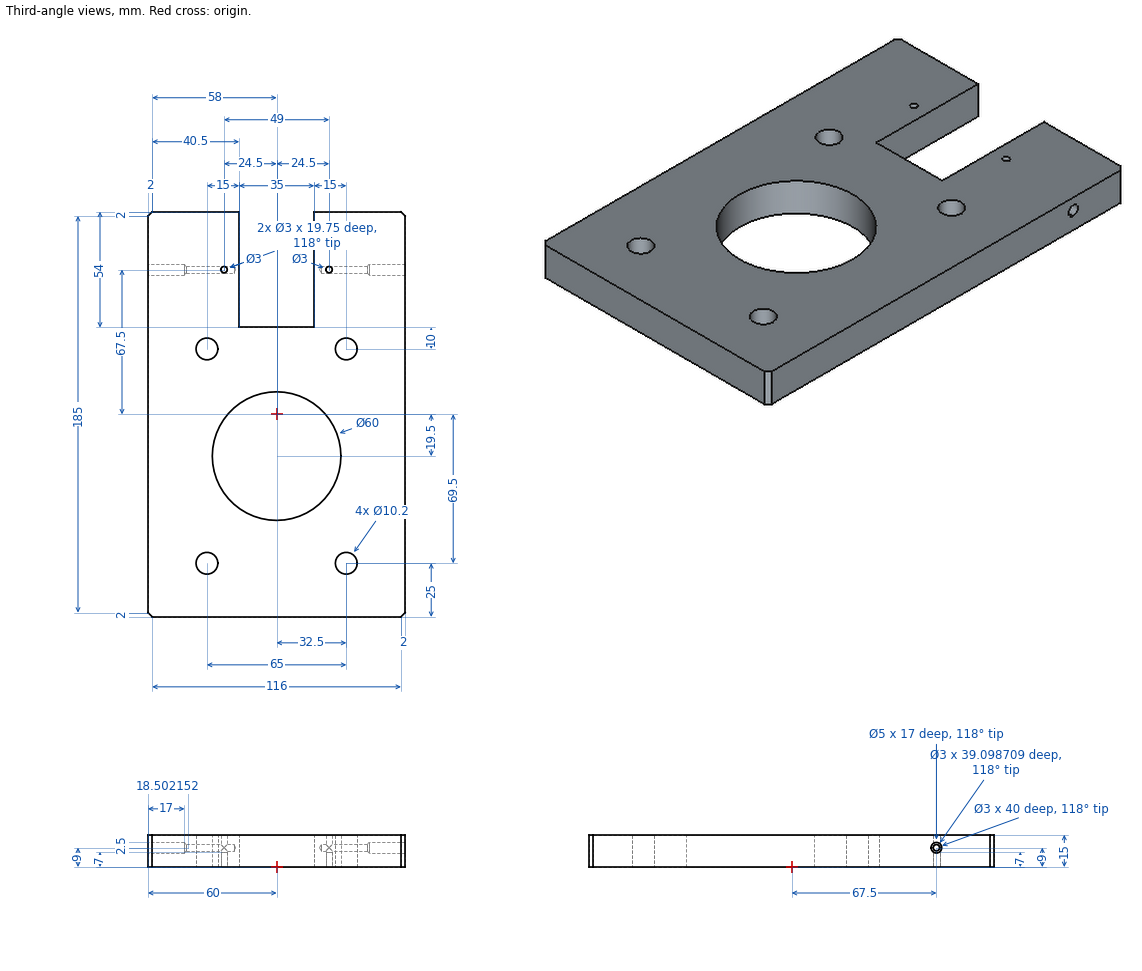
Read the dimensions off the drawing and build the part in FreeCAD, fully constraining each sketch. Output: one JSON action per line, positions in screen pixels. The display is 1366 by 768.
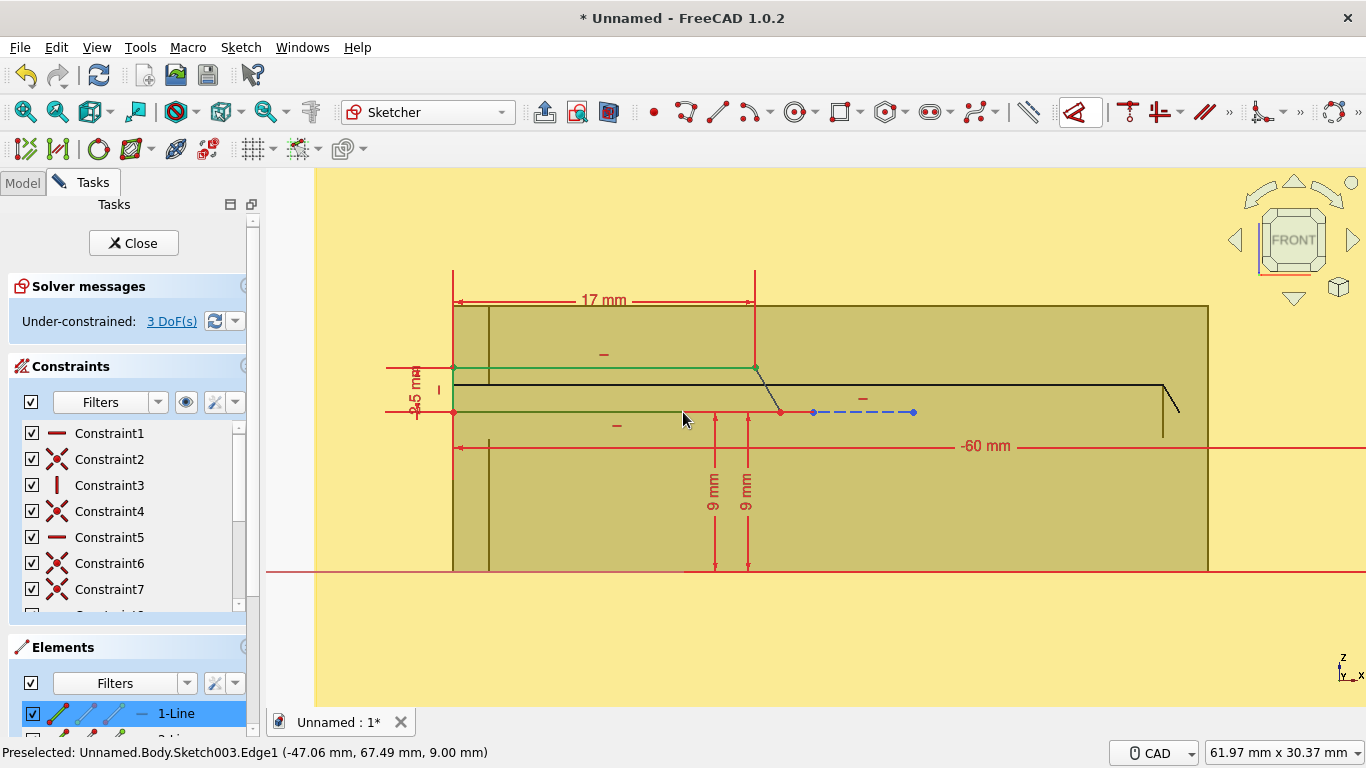
{"action": "key", "text": "l"}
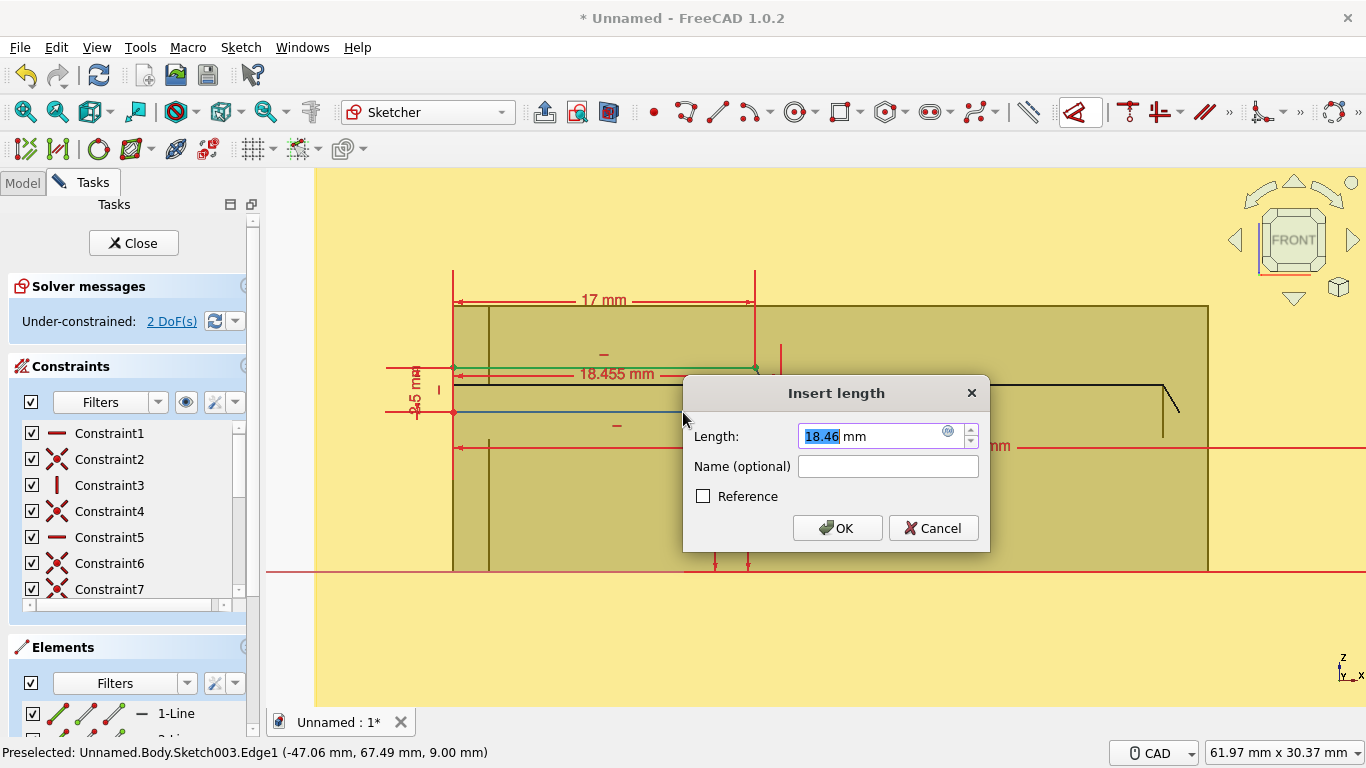
{"action": "type", "text": "18.502152"}
{"action": "key", "text": "Return"}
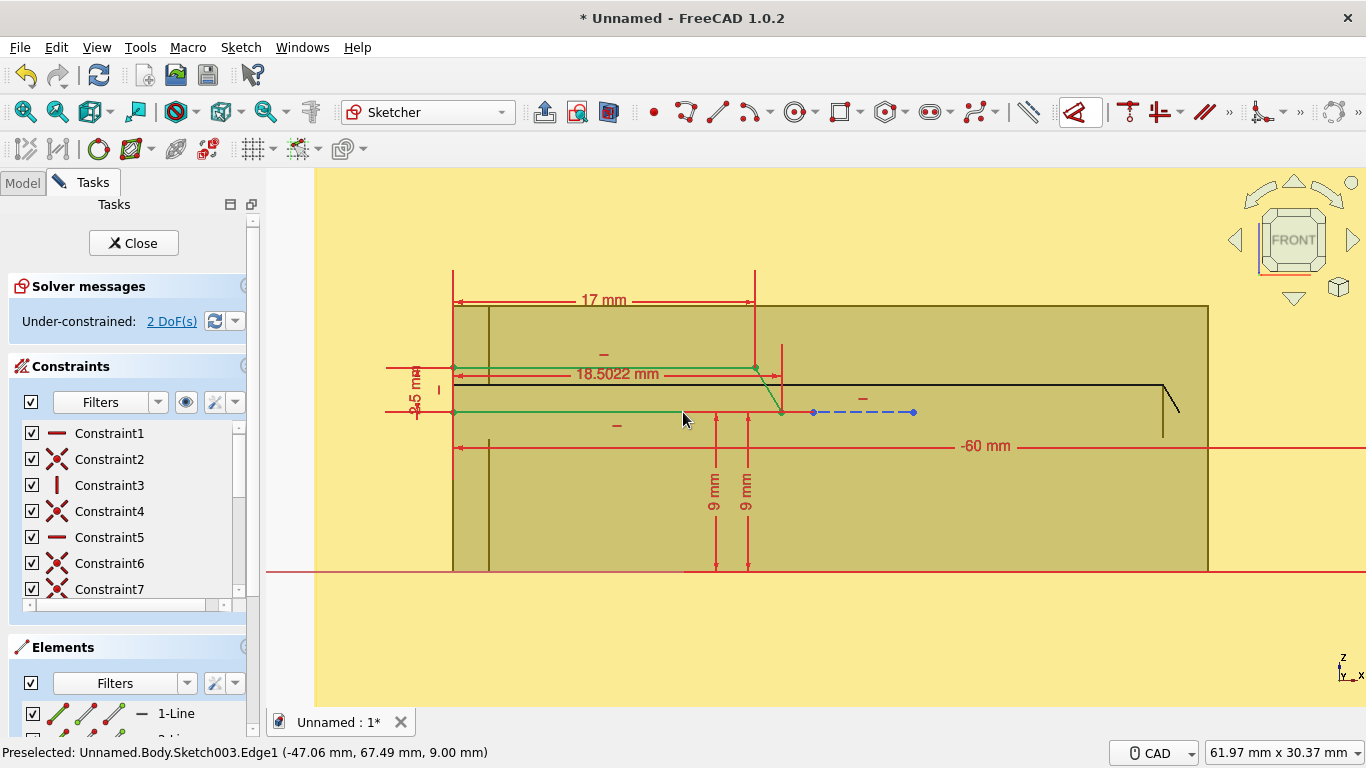
{"action": "left_click", "coordinate": [134, 243]}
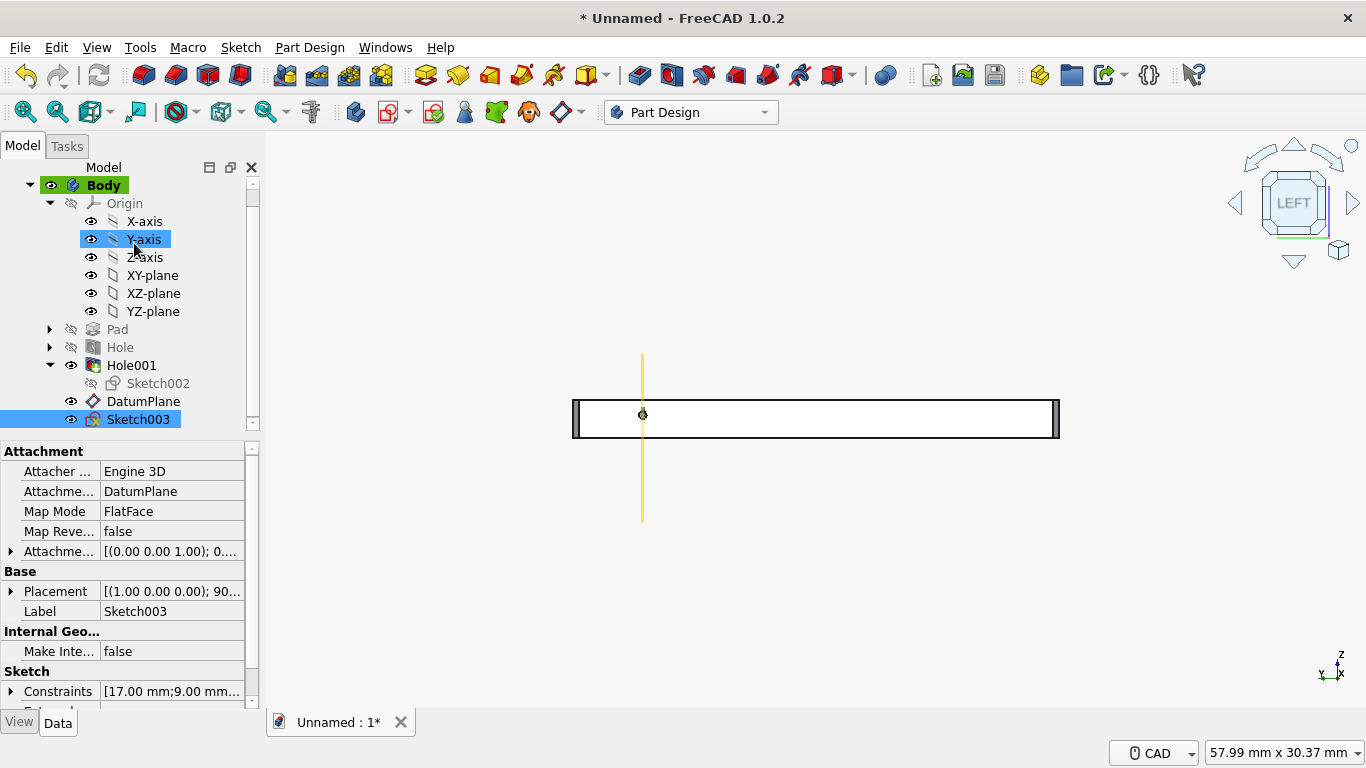
{"action": "left_click", "coordinate": [704, 76]}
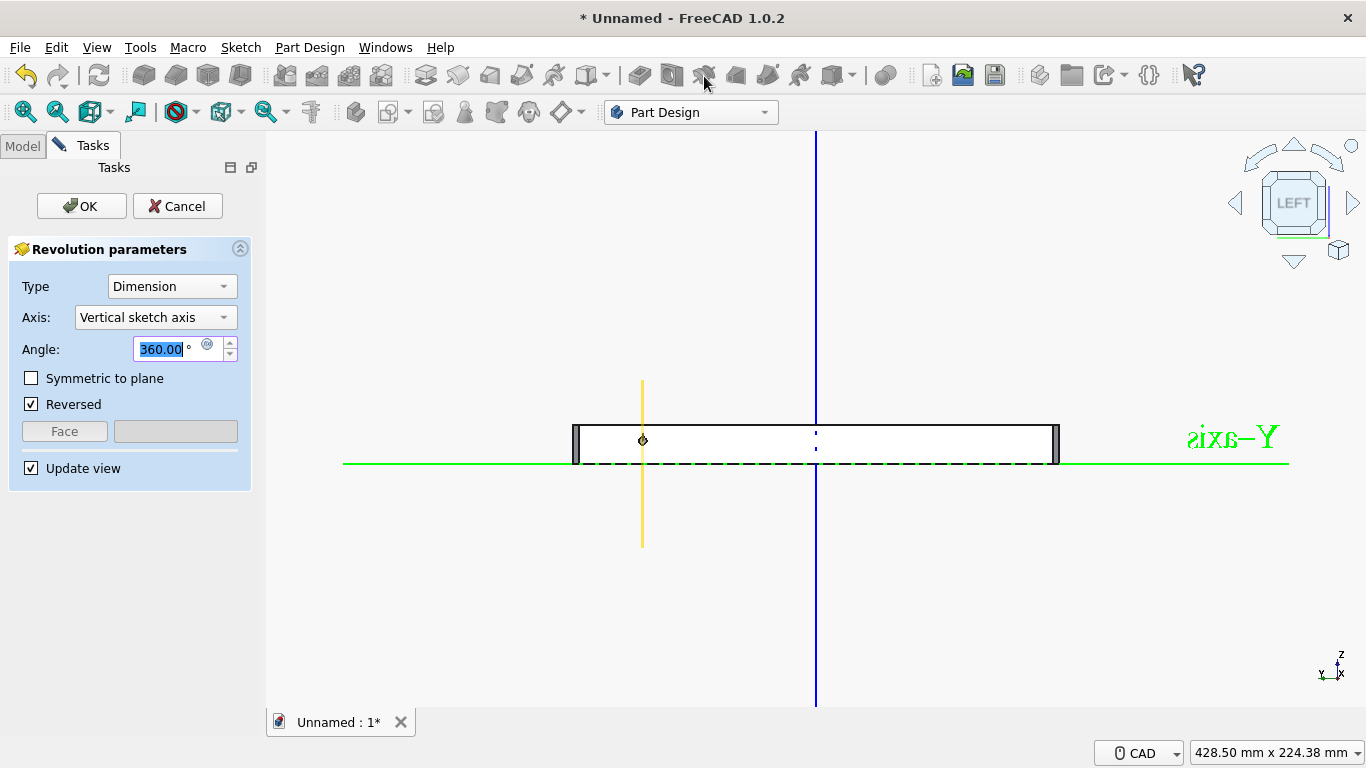
{"action": "left_click", "coordinate": [156, 318]}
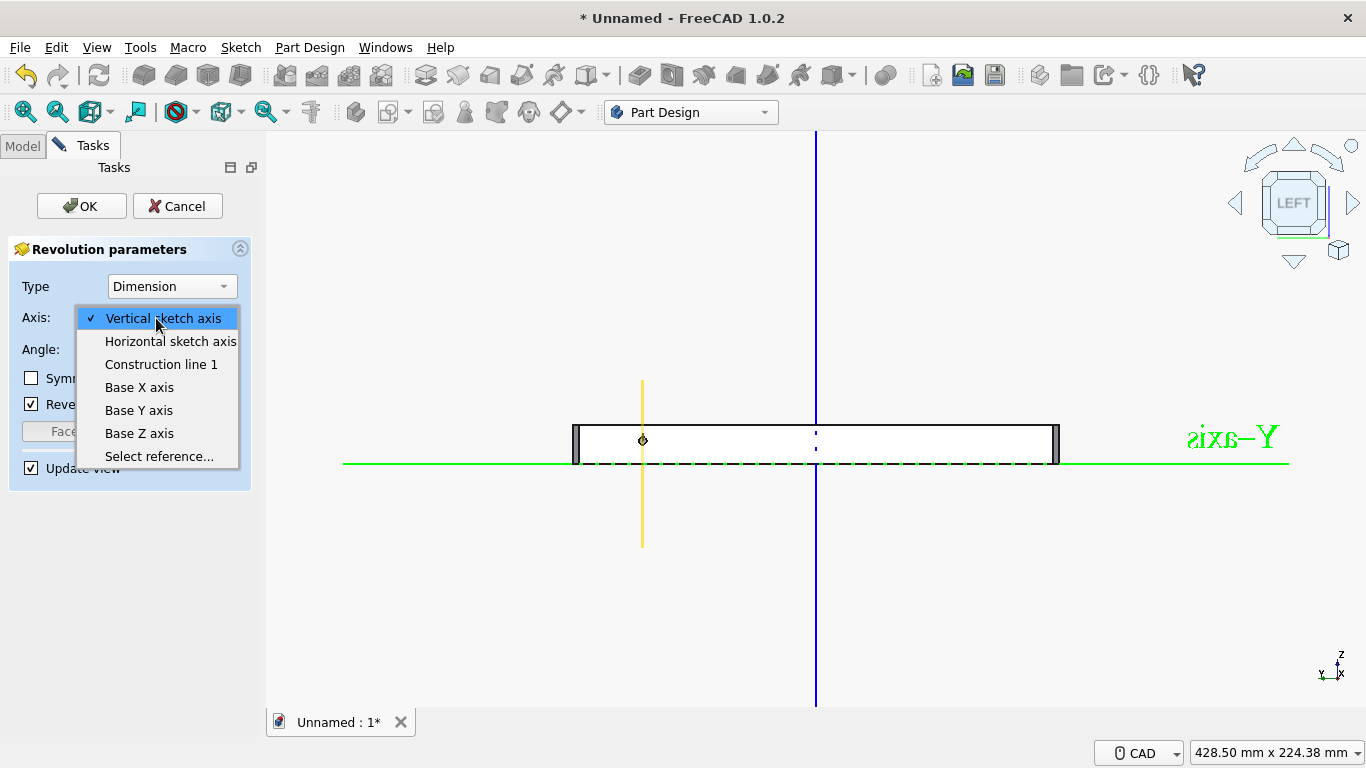
{"action": "left_click", "coordinate": [156, 364]}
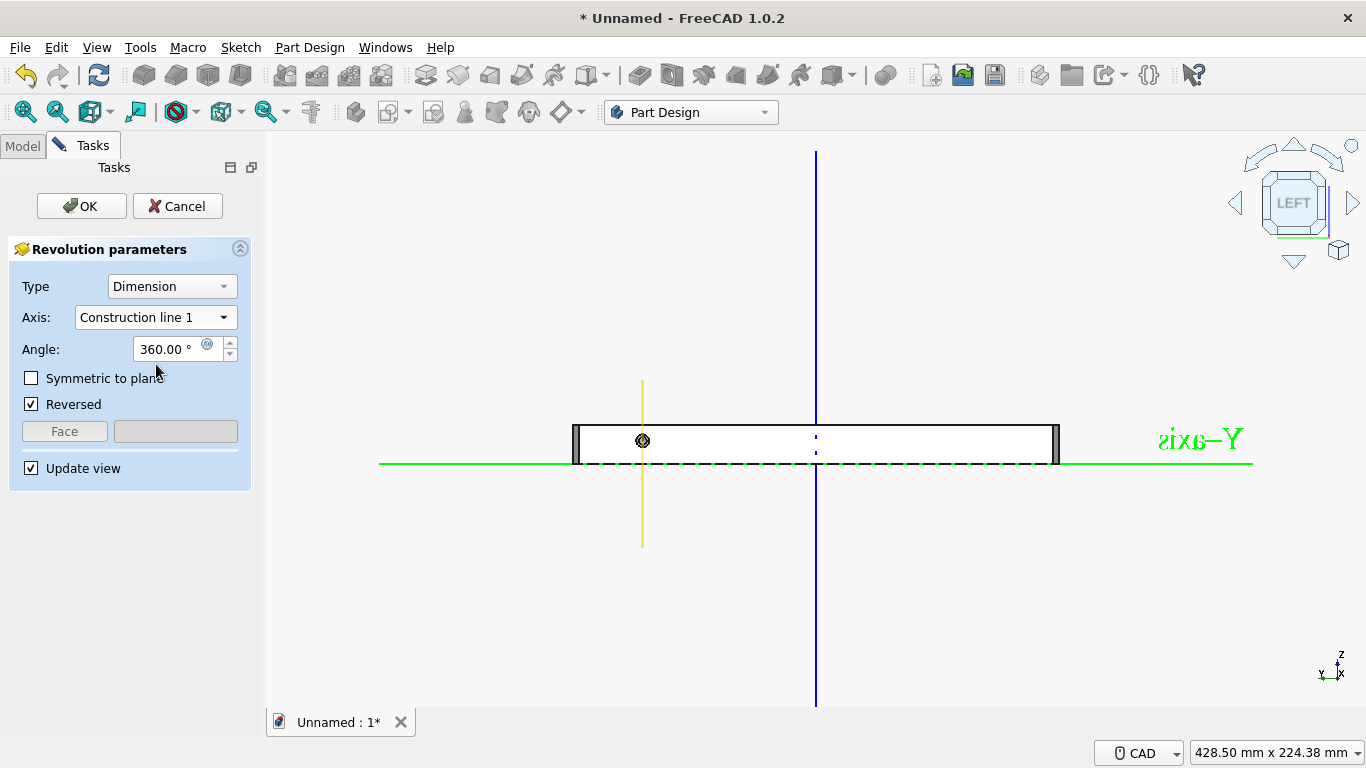
{"action": "left_click", "coordinate": [82, 206]}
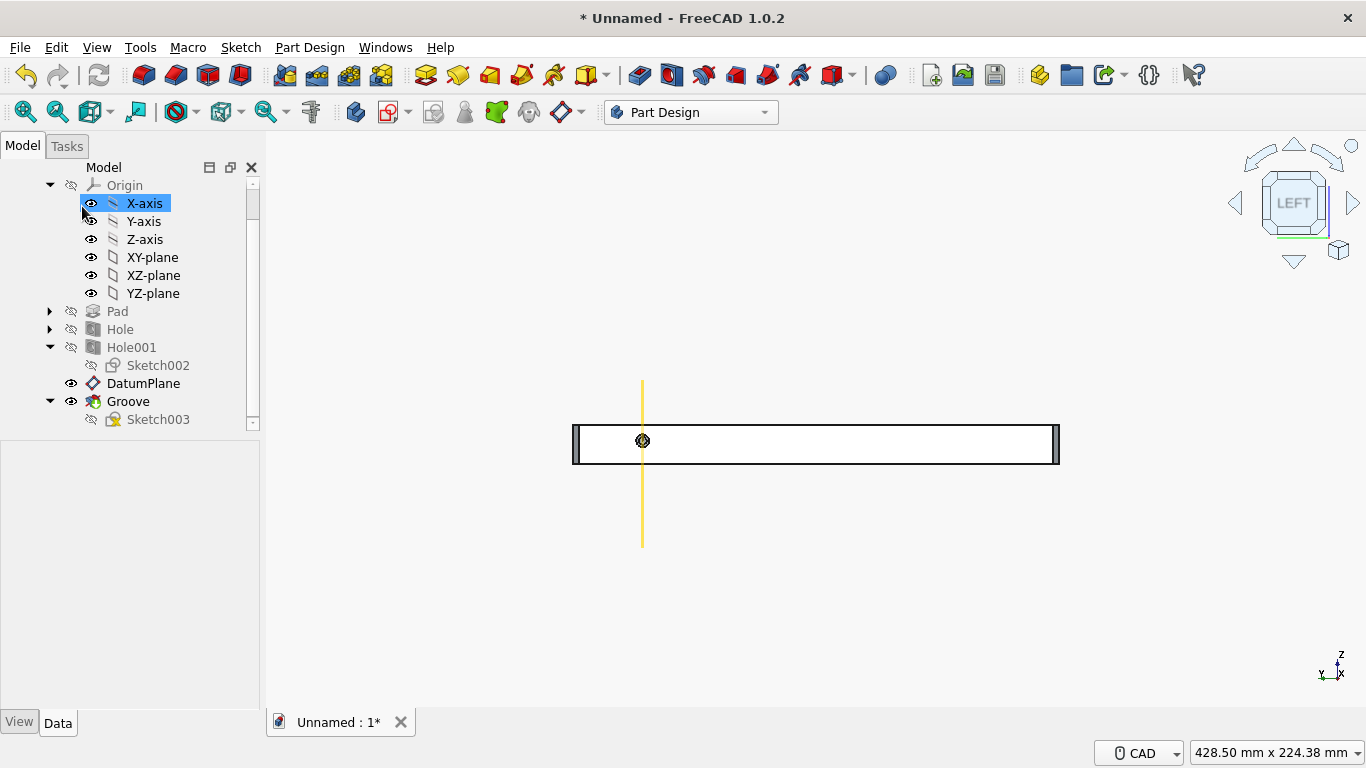
{"action": "left_click", "coordinate": [116, 383]}
{"action": "key", "text": "space"}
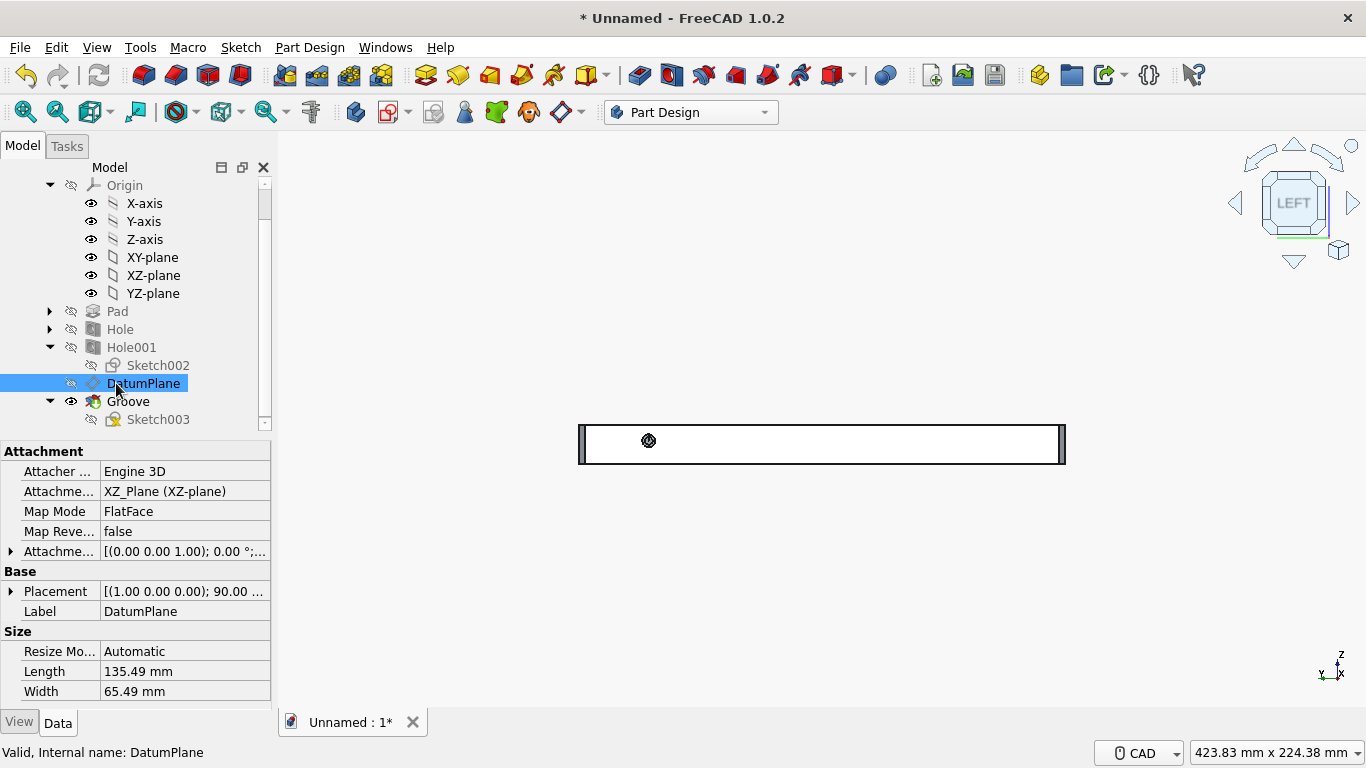
{"action": "key", "text": "v f"}